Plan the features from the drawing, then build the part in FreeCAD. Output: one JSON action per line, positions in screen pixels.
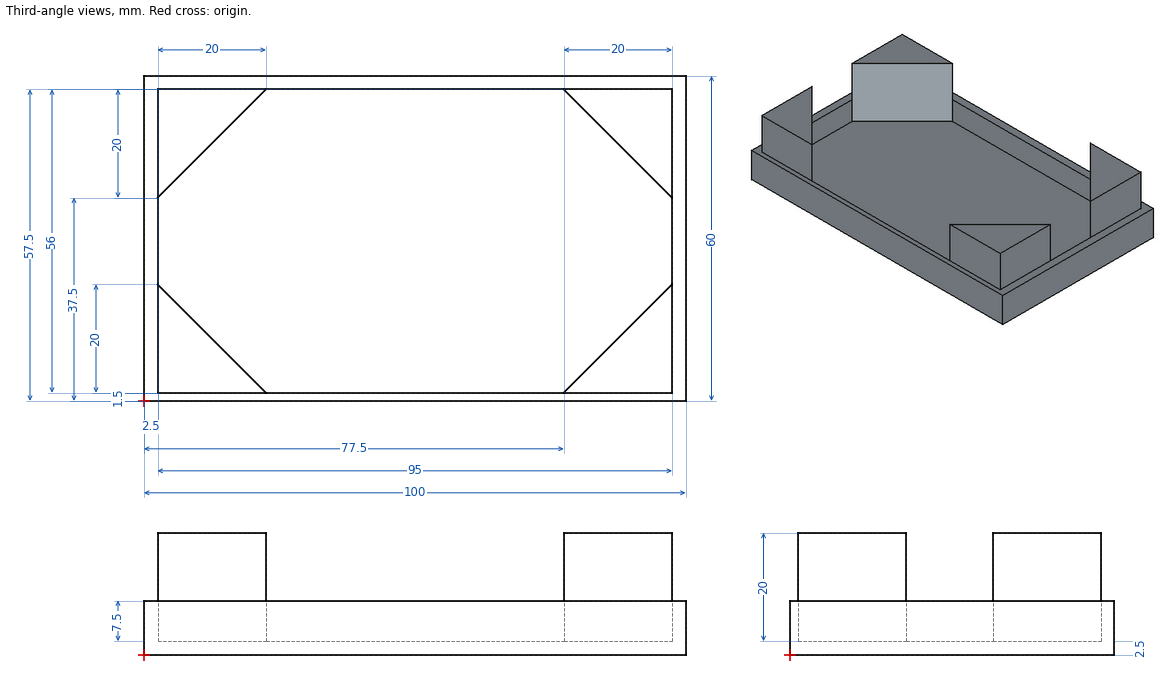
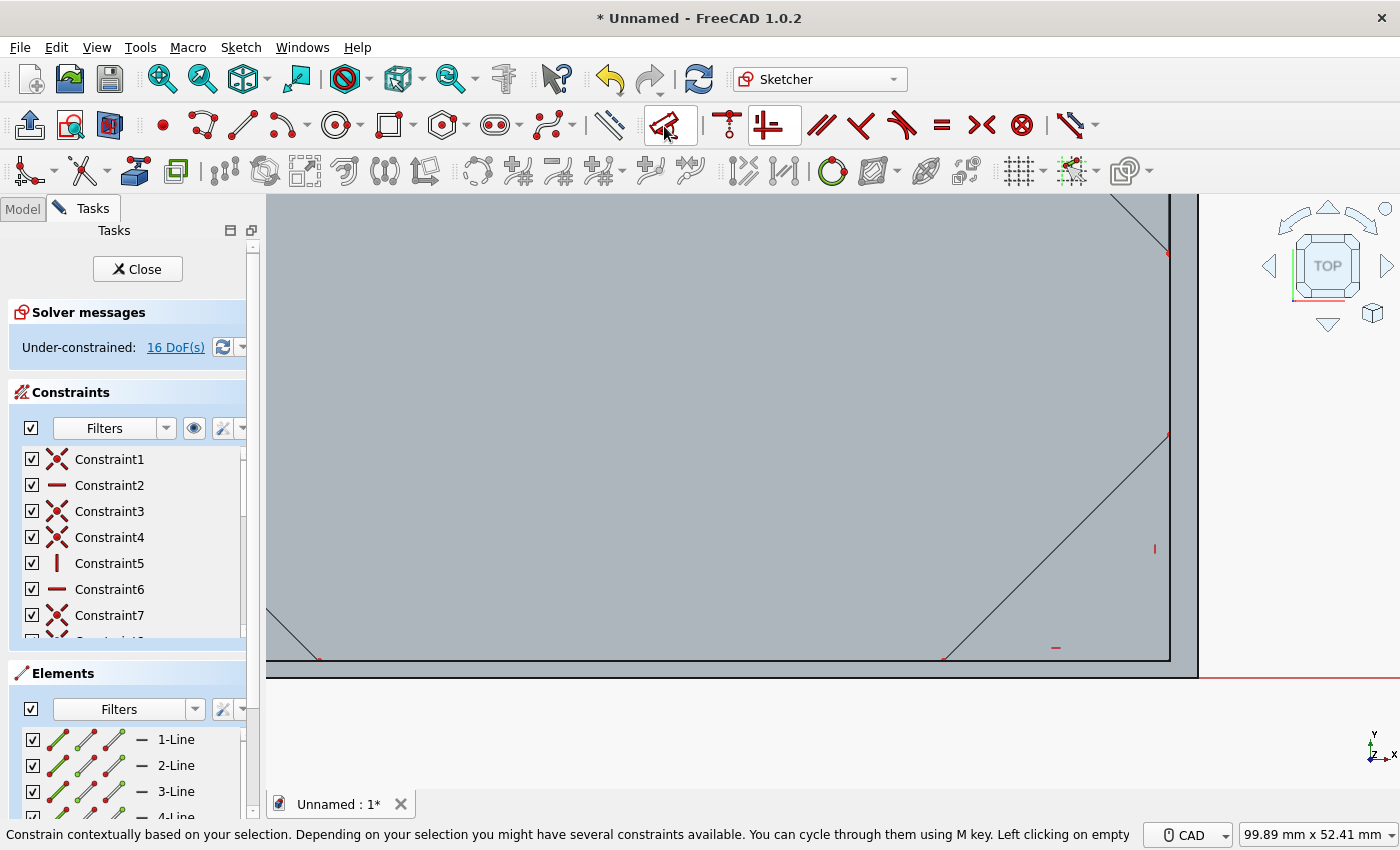
{"action": "scroll", "coordinate": [944, 662], "scroll_direction": "down", "scroll_amount": 3}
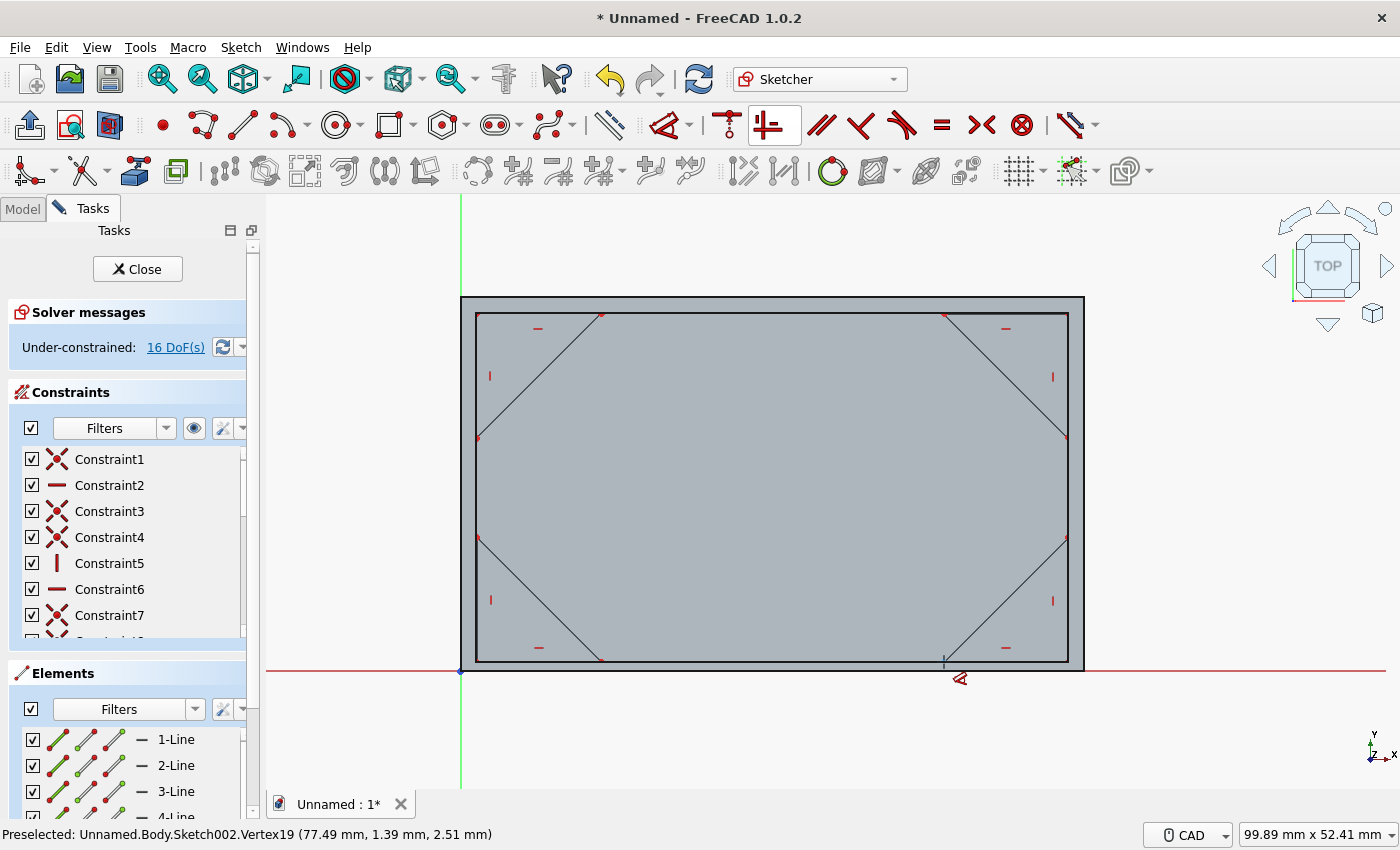
{"action": "left_click", "coordinate": [564, 313]}
{"action": "left_click", "coordinate": [539, 279]}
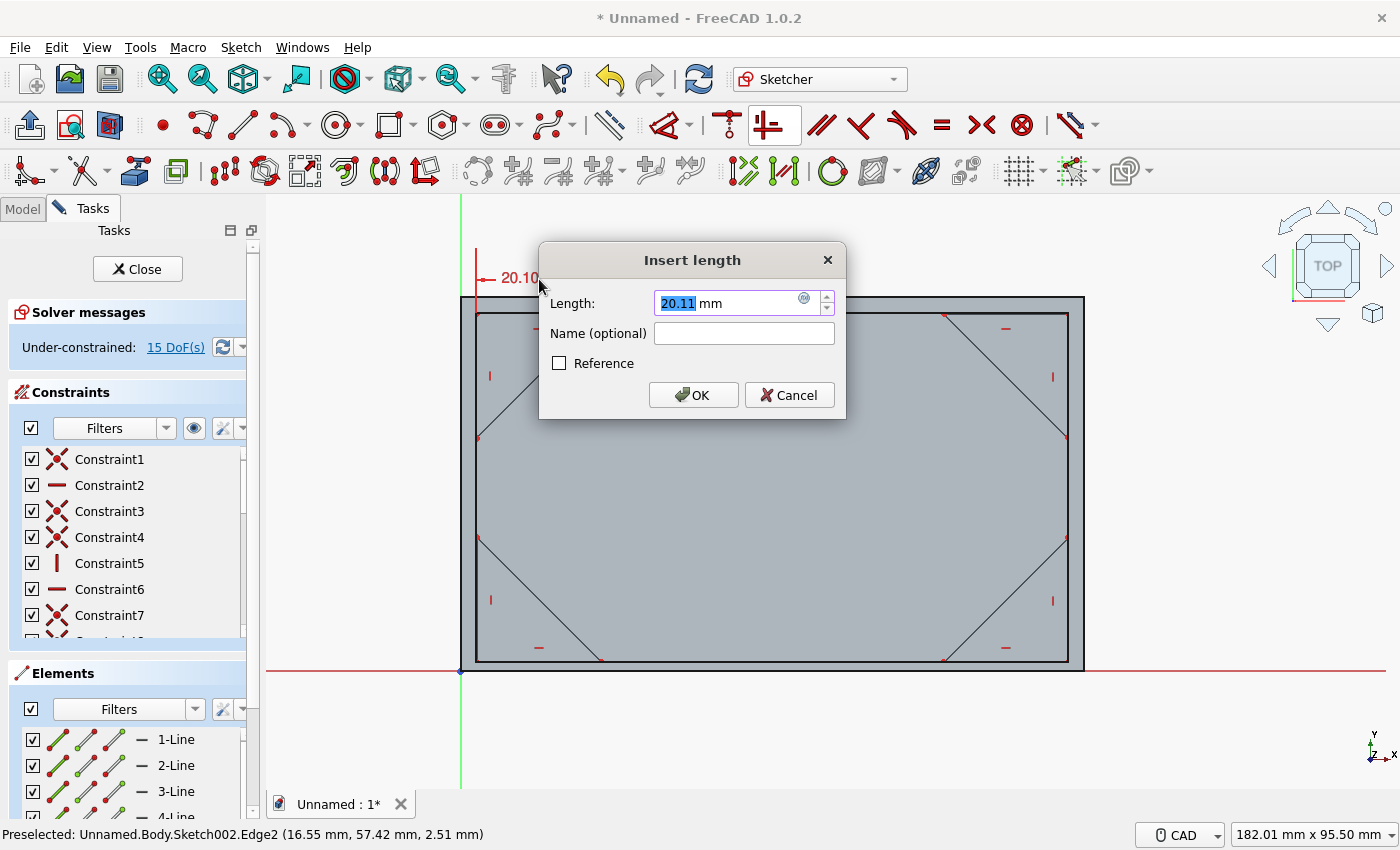
{"action": "type", "text": "20"}
{"action": "key", "text": "Return"}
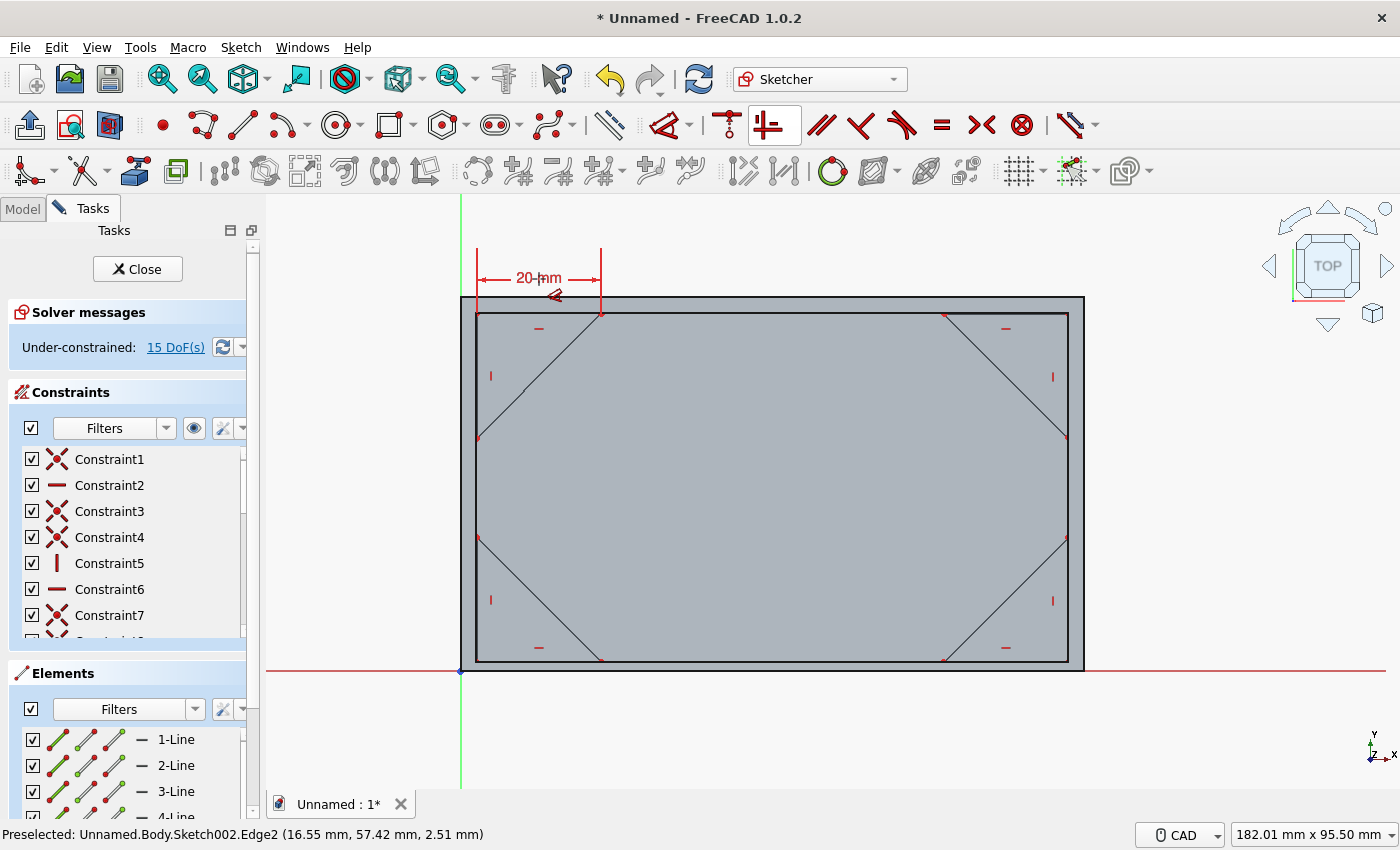
{"action": "left_click", "coordinate": [477, 351]}
{"action": "left_click", "coordinate": [443, 376]}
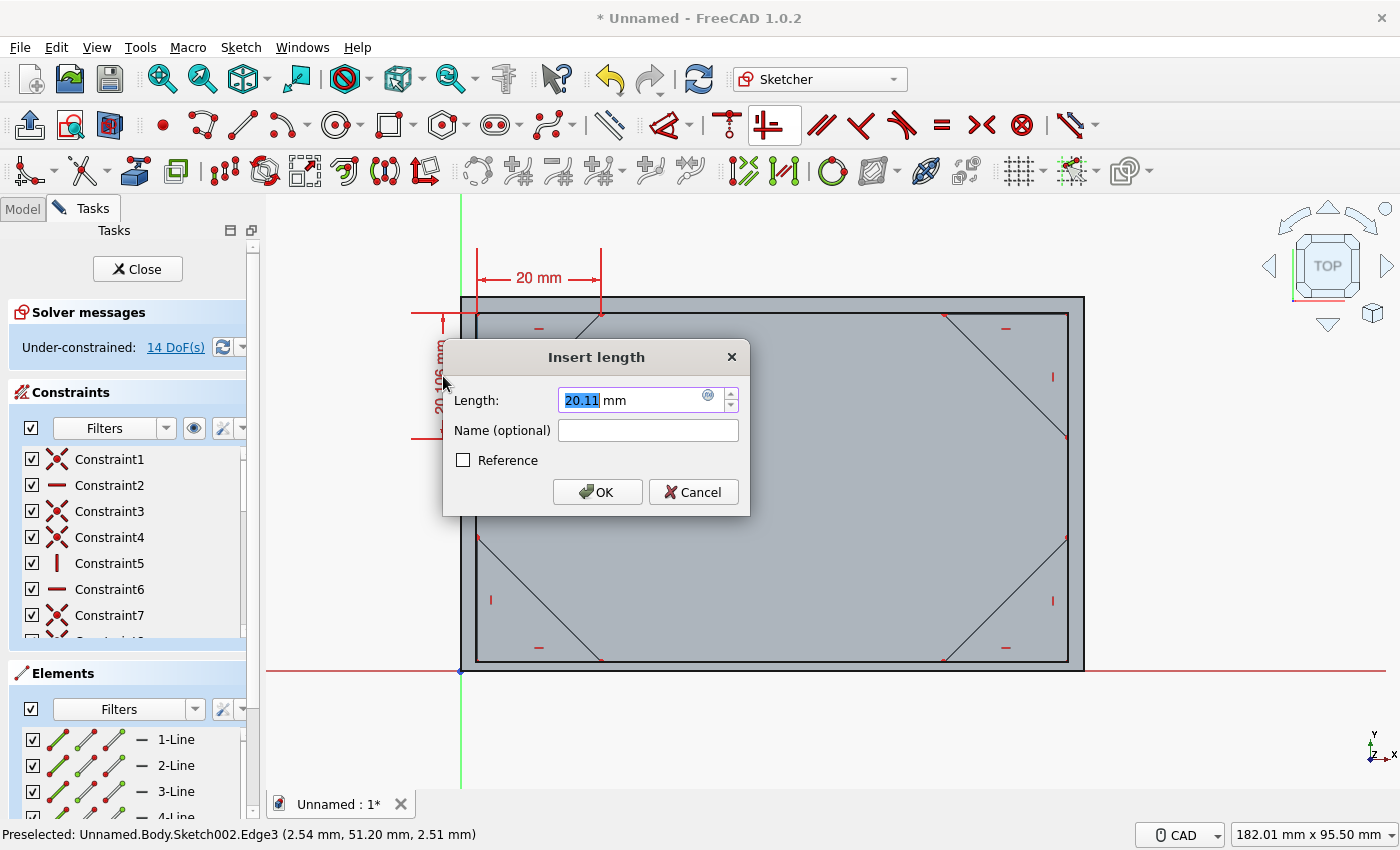
{"action": "type", "text": "20"}
{"action": "key", "text": "Return"}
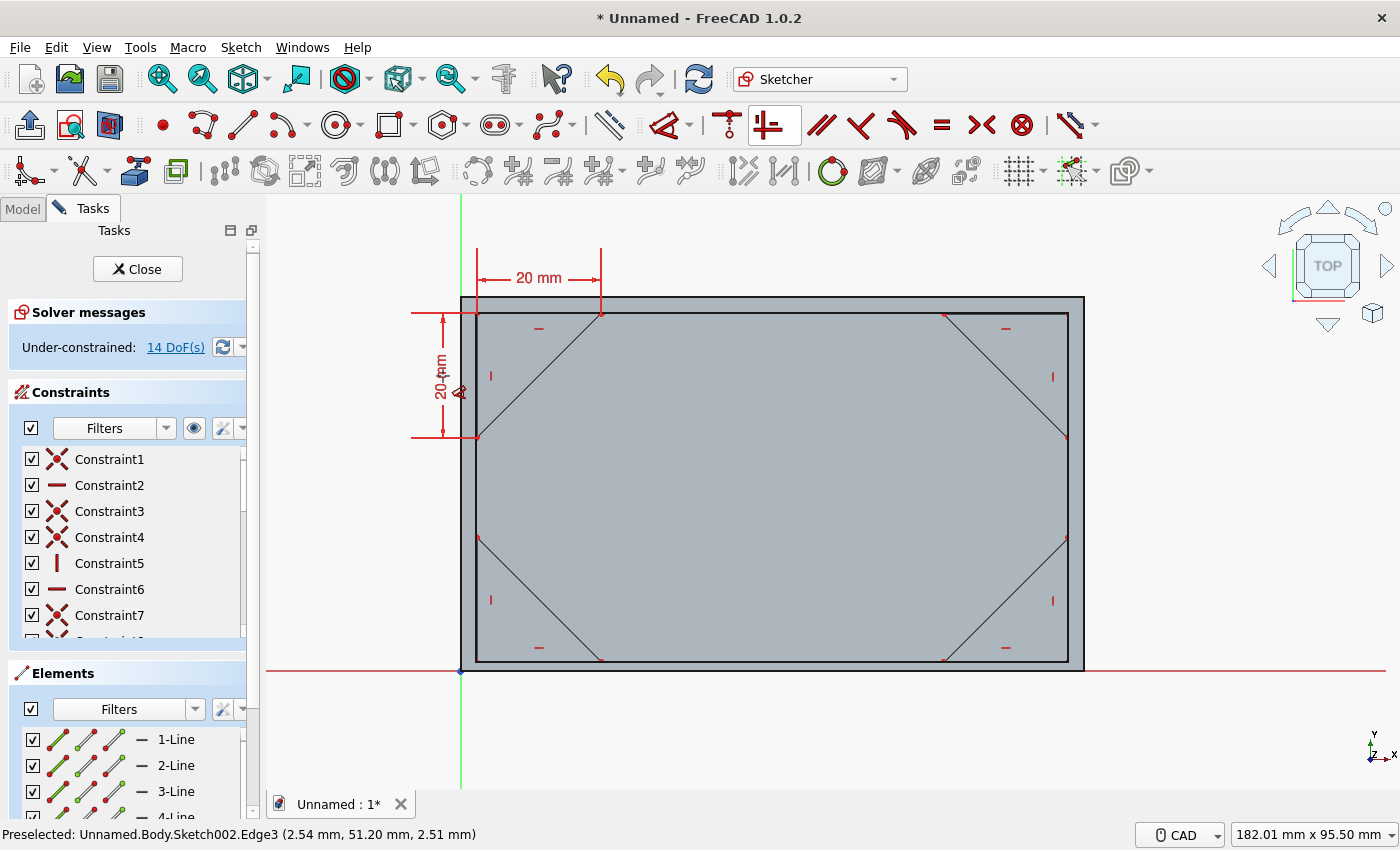
{"action": "scroll", "coordinate": [514, 662], "scroll_direction": "up", "scroll_amount": 3}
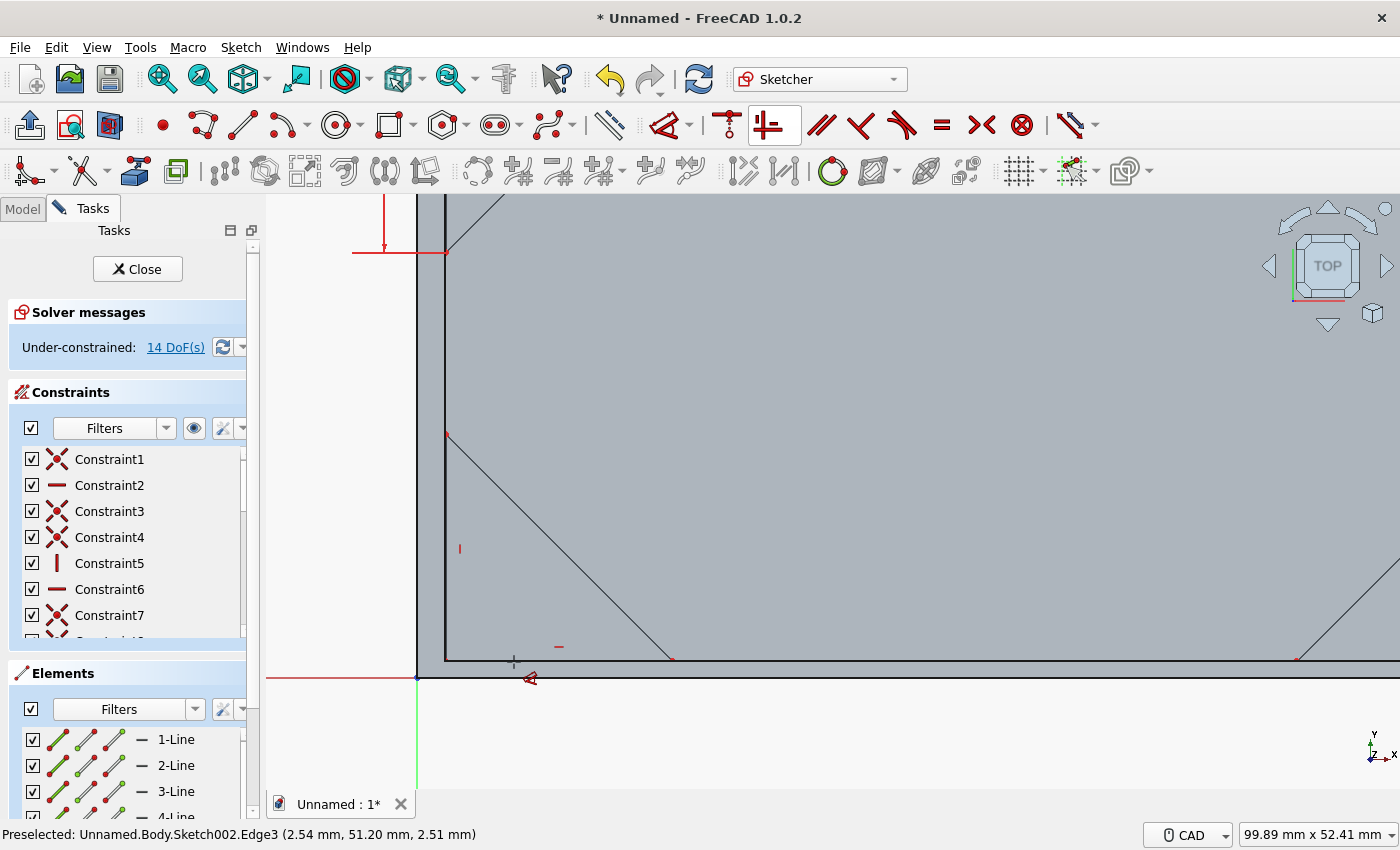
{"action": "left_click", "coordinate": [514, 662]}
{"action": "left_click", "coordinate": [559, 696]}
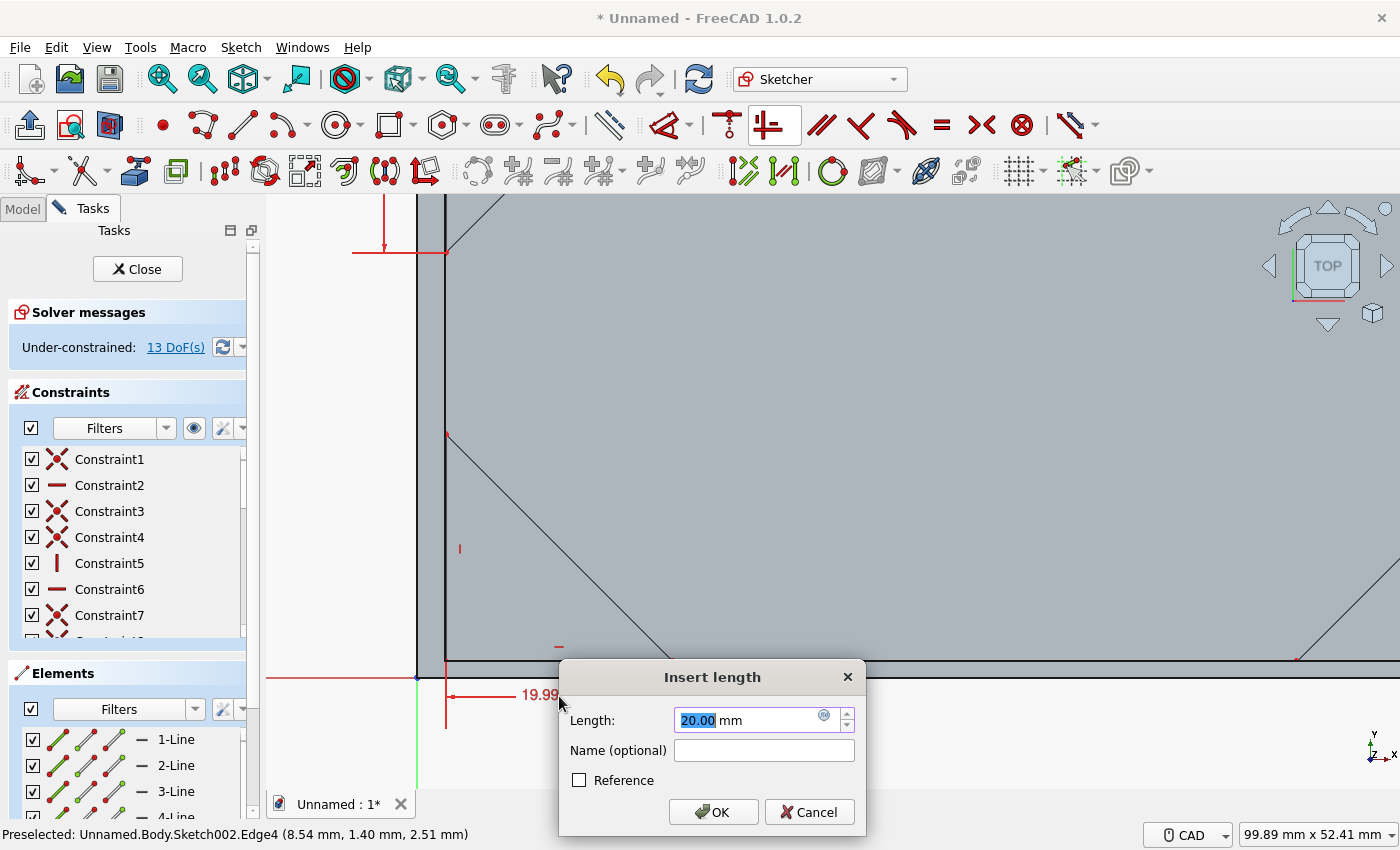
{"action": "type", "text": "20"}
{"action": "key", "text": "Return"}